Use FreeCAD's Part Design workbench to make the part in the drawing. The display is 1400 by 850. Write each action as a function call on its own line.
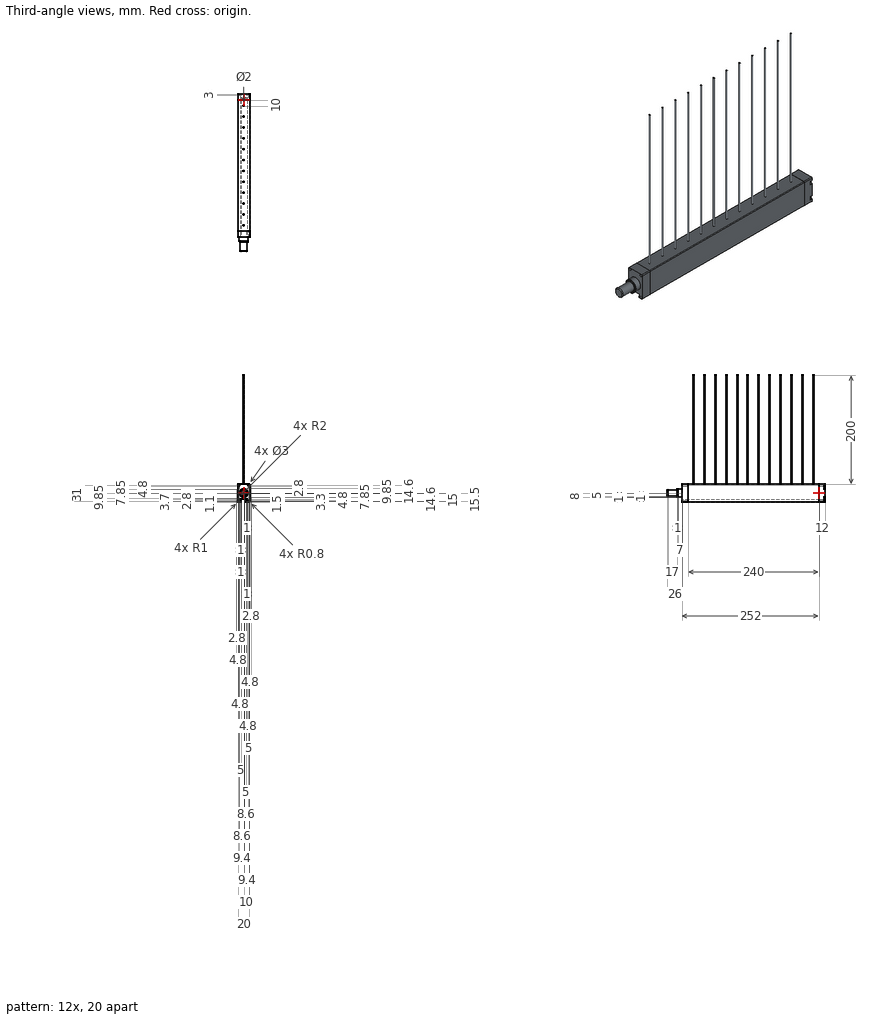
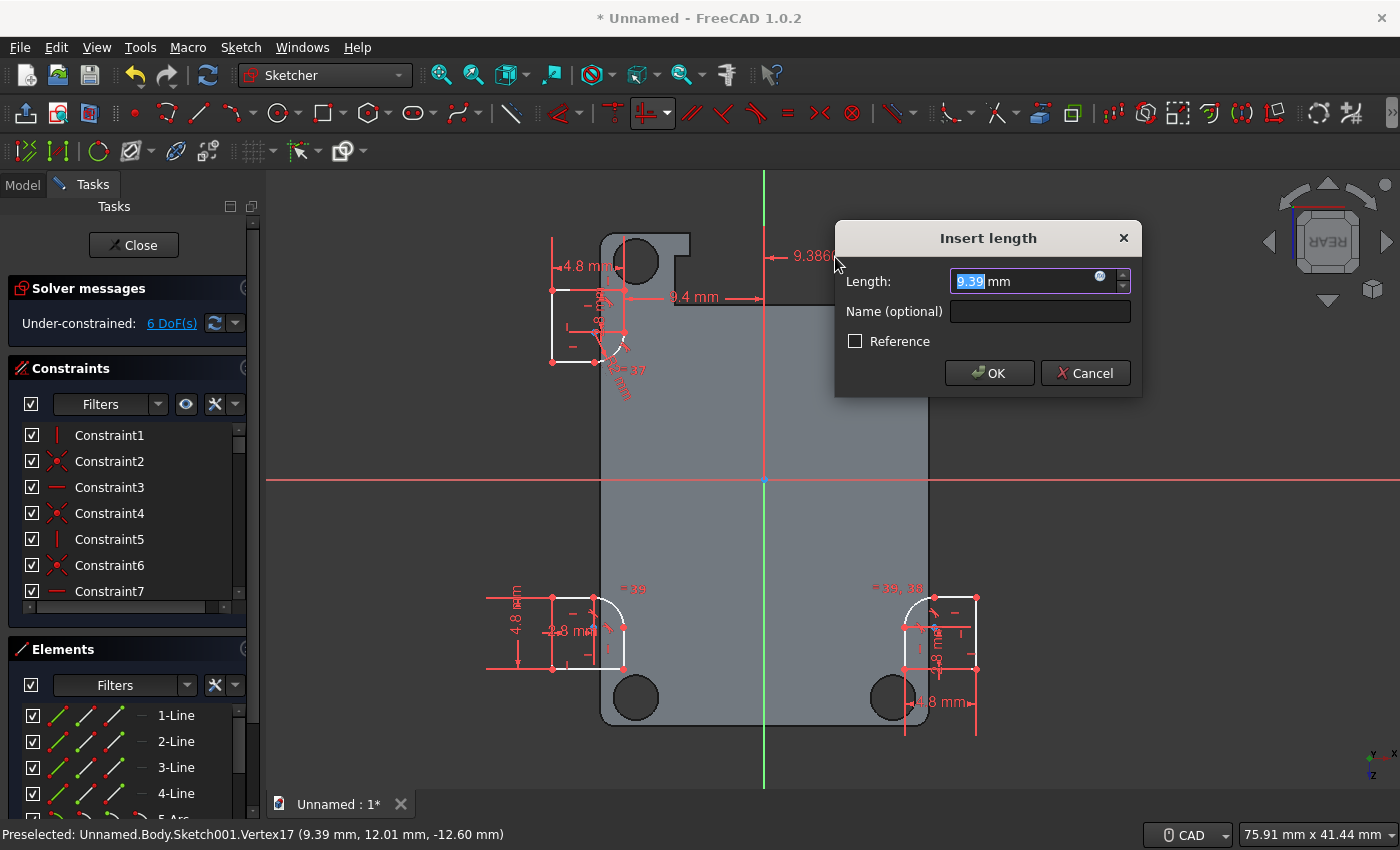
text(9.4)
key(Return)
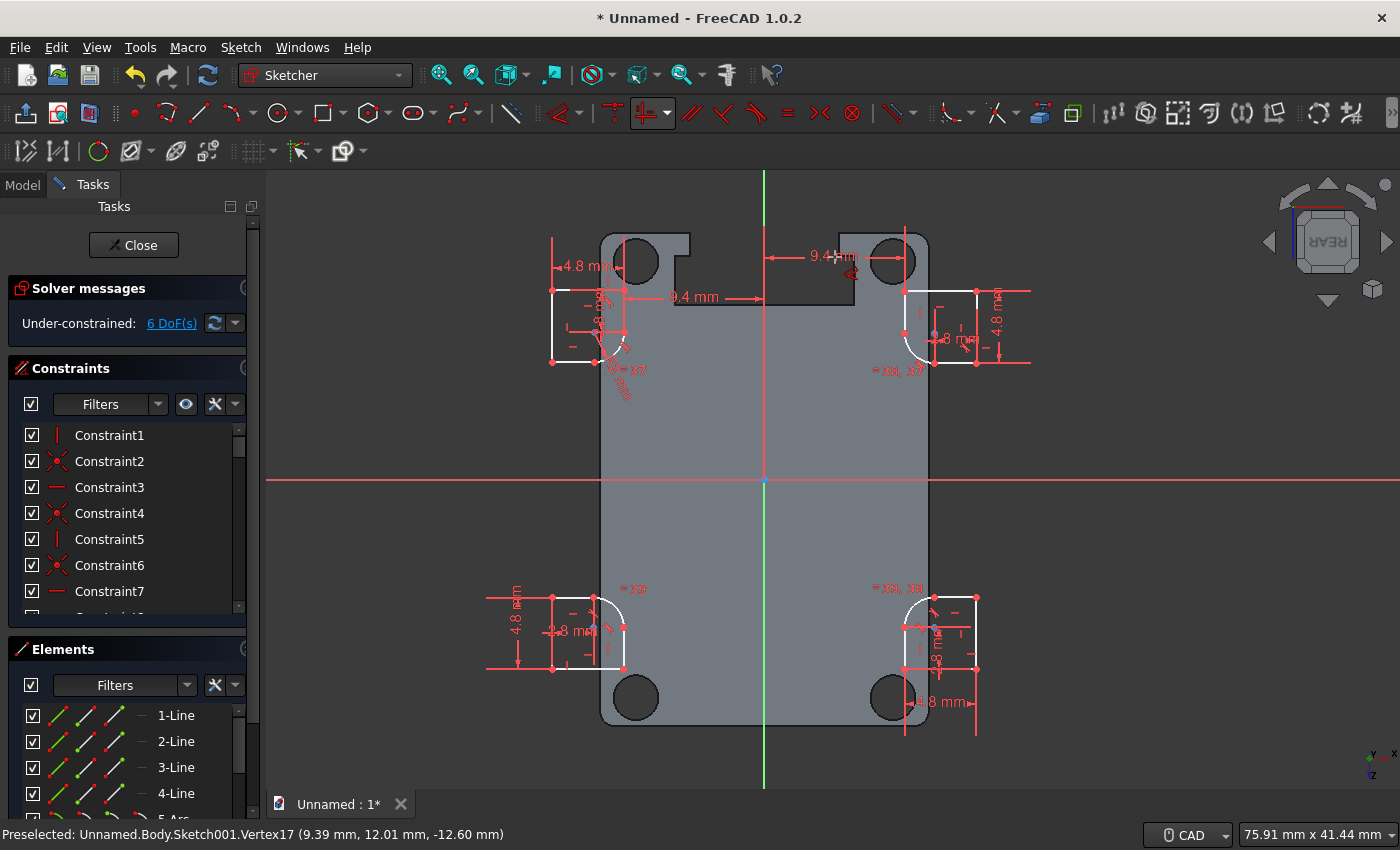
click(905, 627)
click(835, 661)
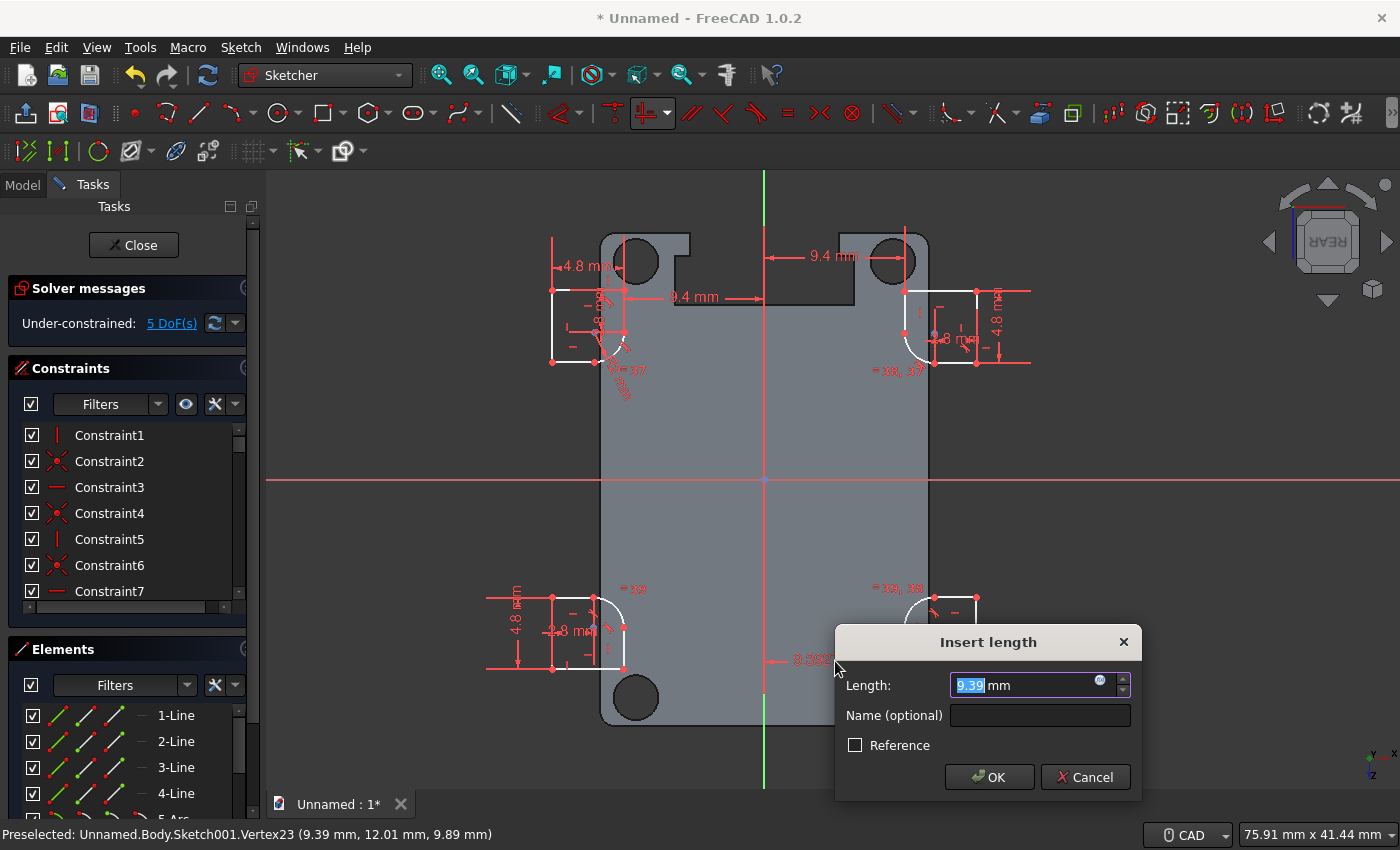
text(9.4)
key(Return)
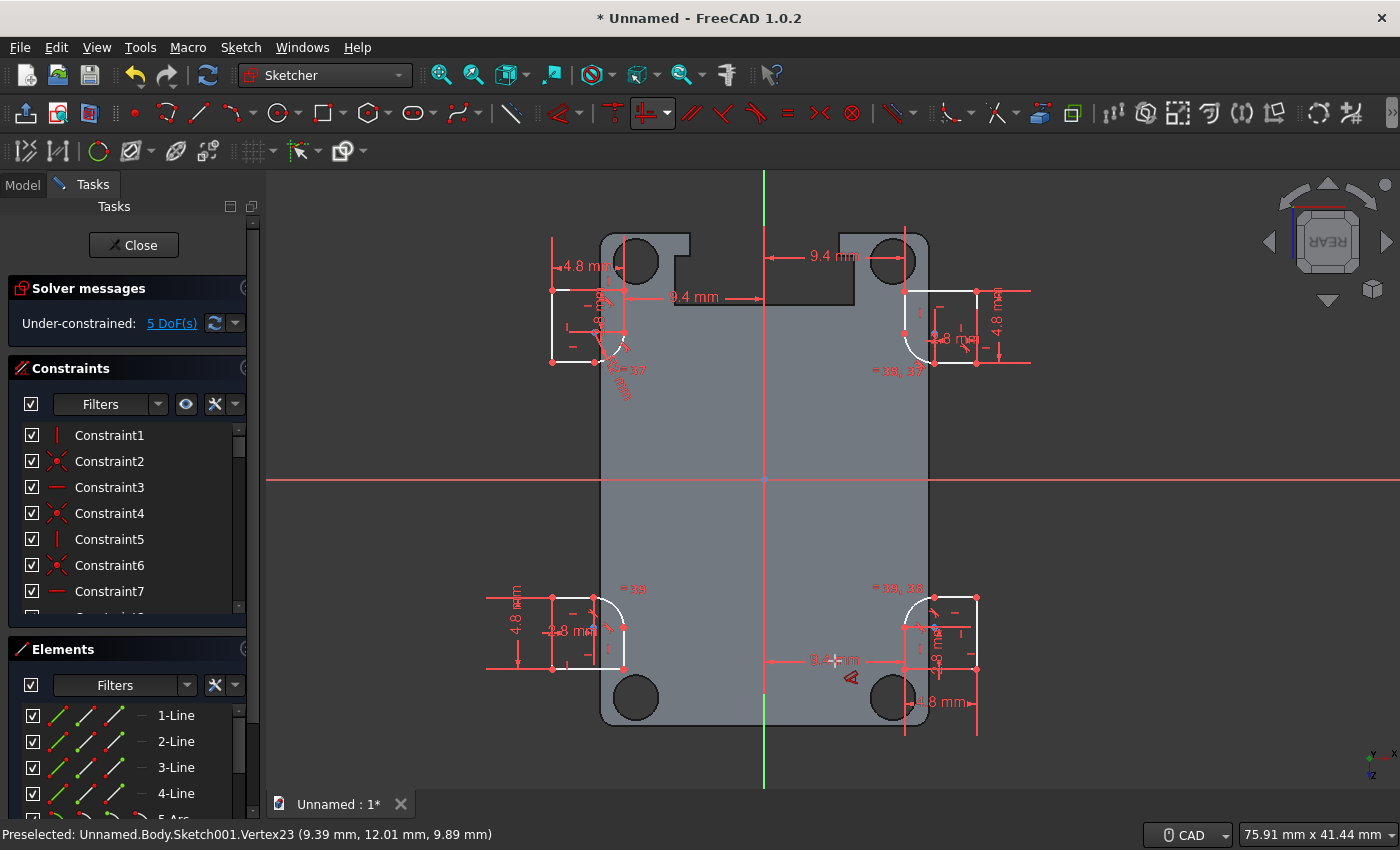
click(624, 669)
click(694, 703)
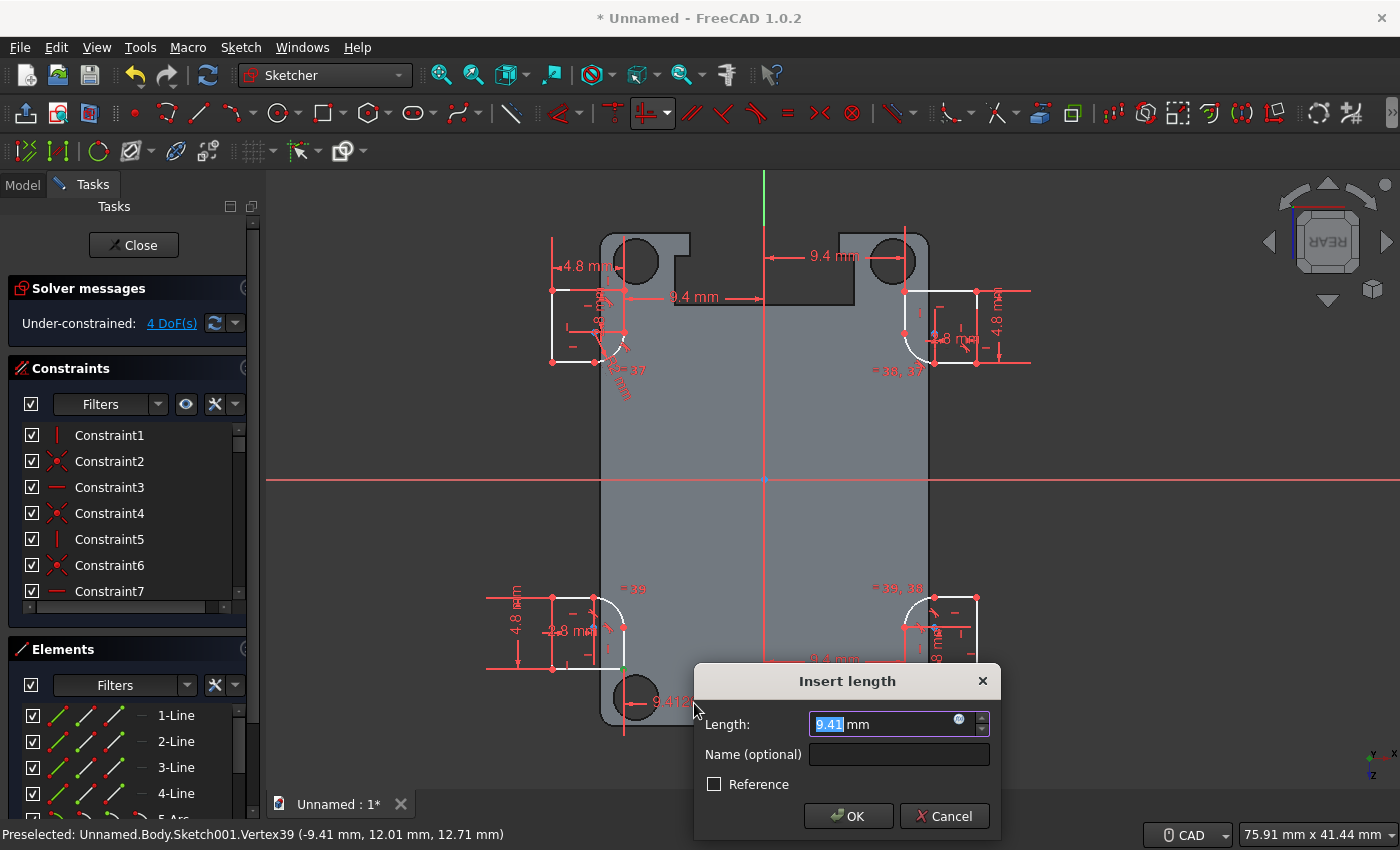
text(9.4)
key(Return)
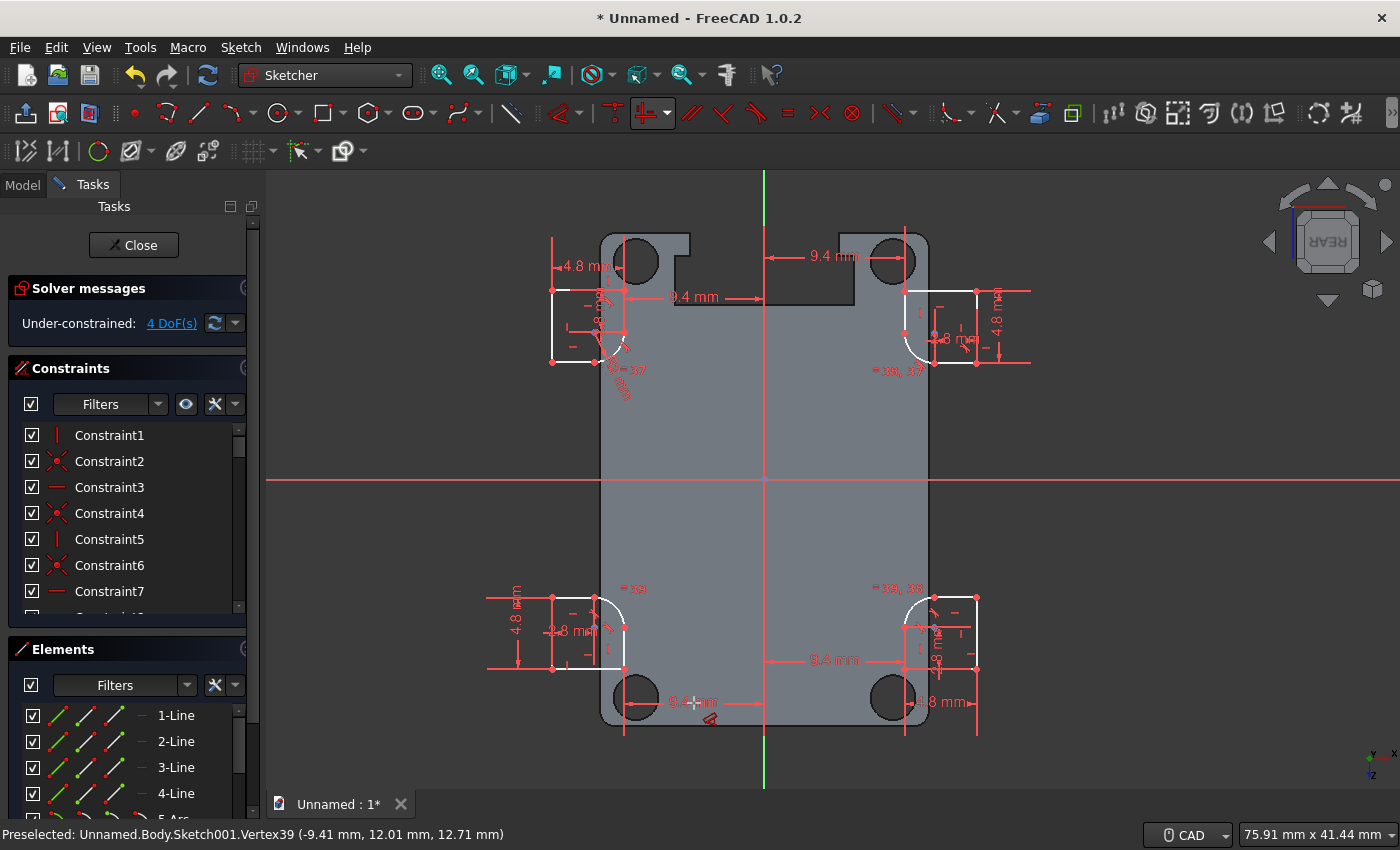
click(624, 332)
click(590, 406)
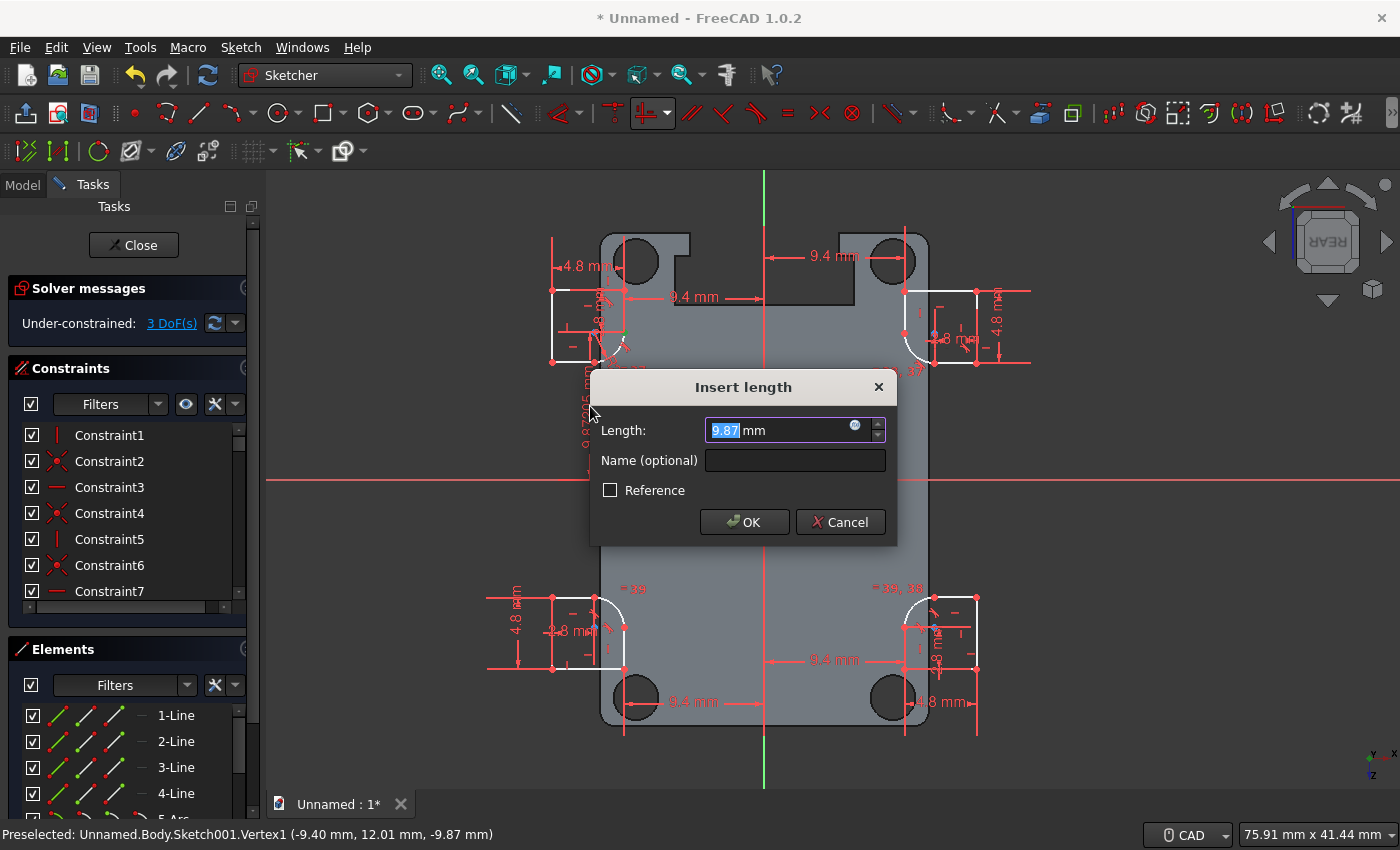
text(9.85)
key(Return)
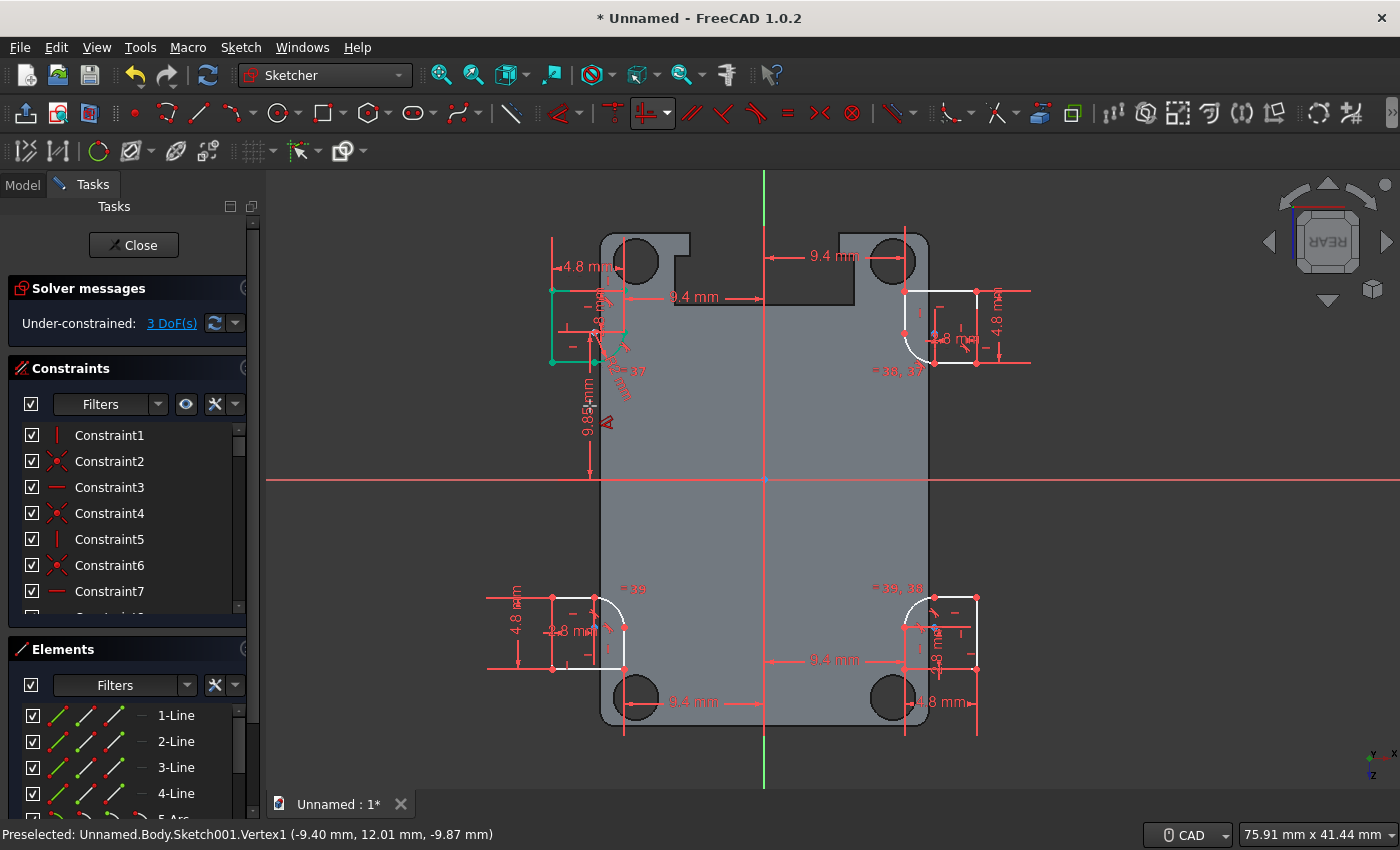
click(935, 363)
click(969, 421)